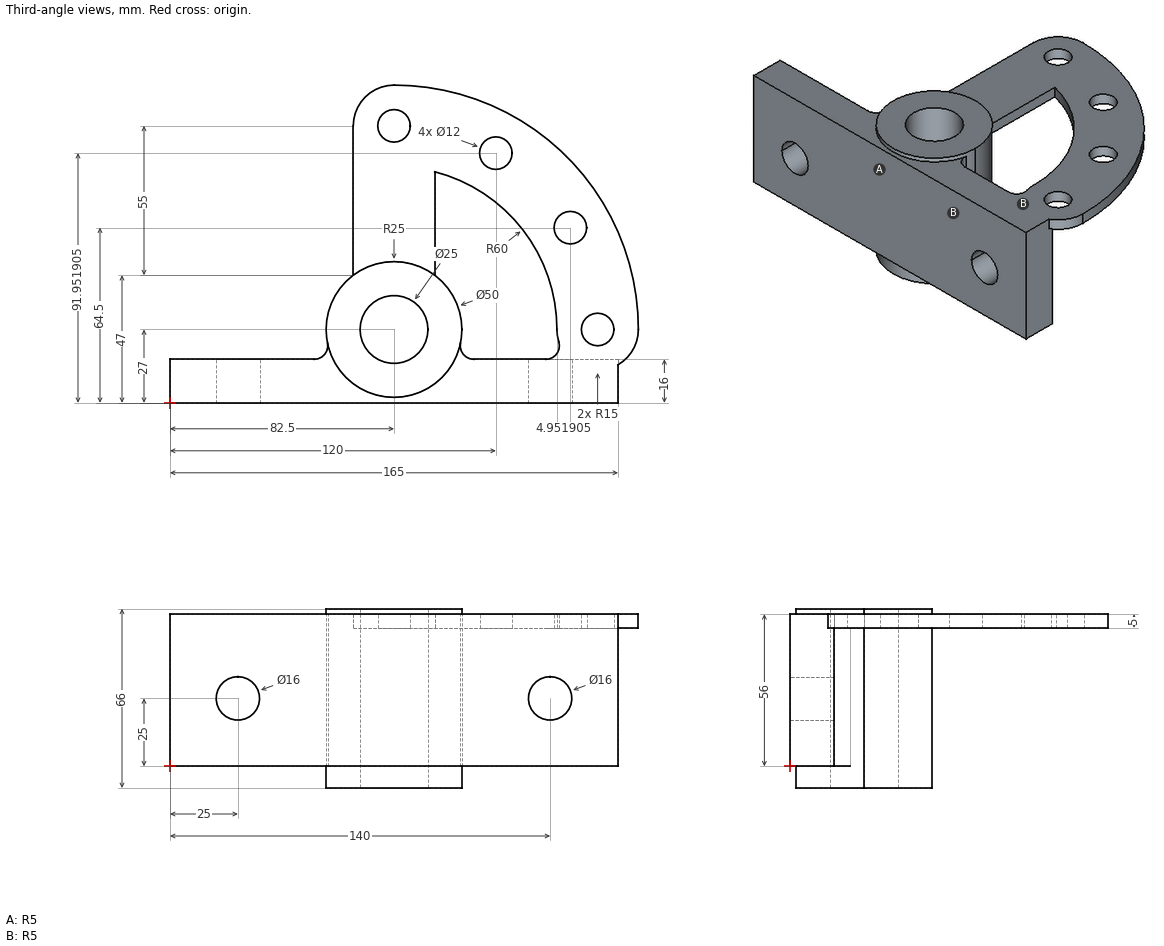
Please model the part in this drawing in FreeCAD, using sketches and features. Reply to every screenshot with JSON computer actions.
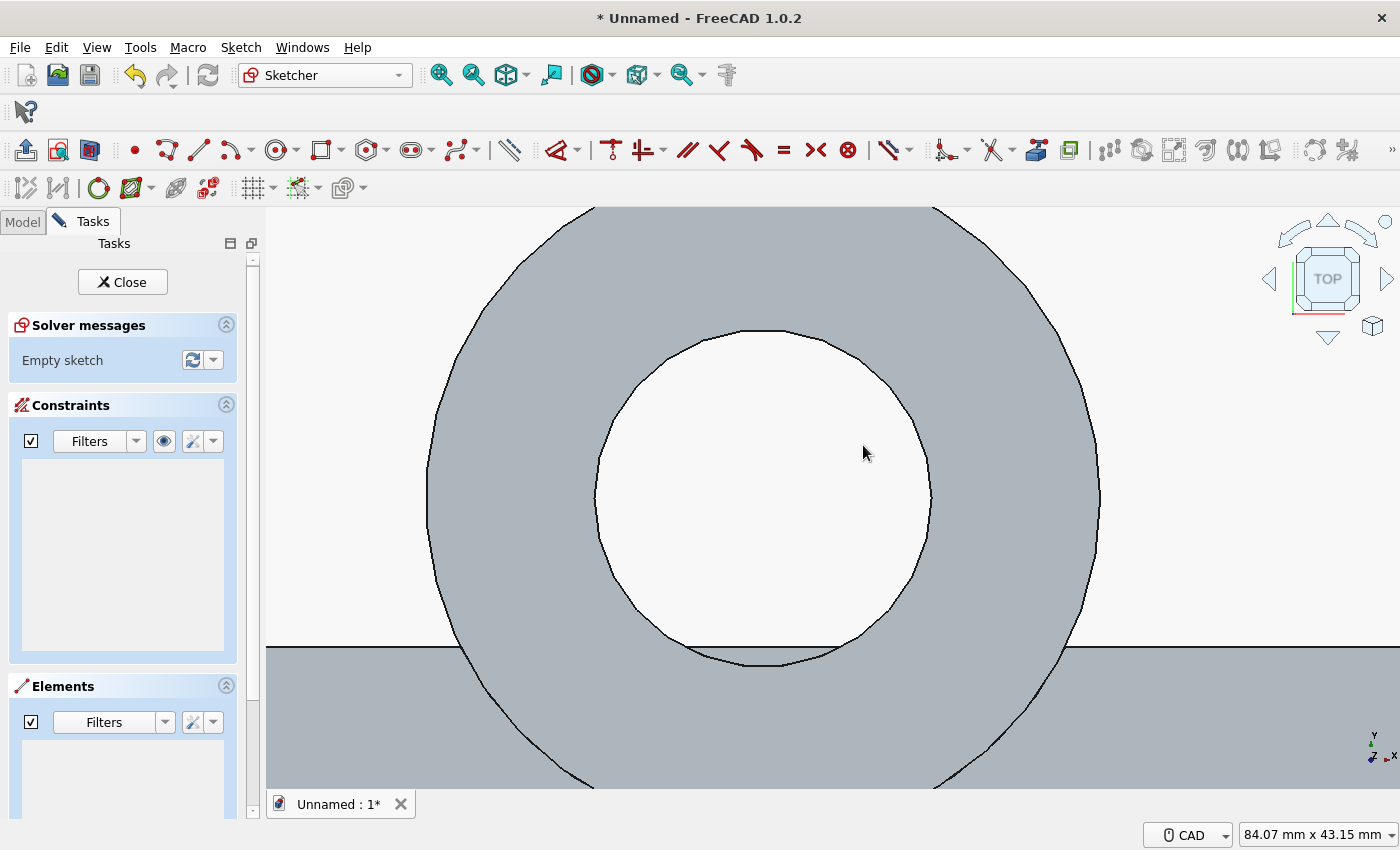
{"action": "left_click", "coordinate": [276, 150]}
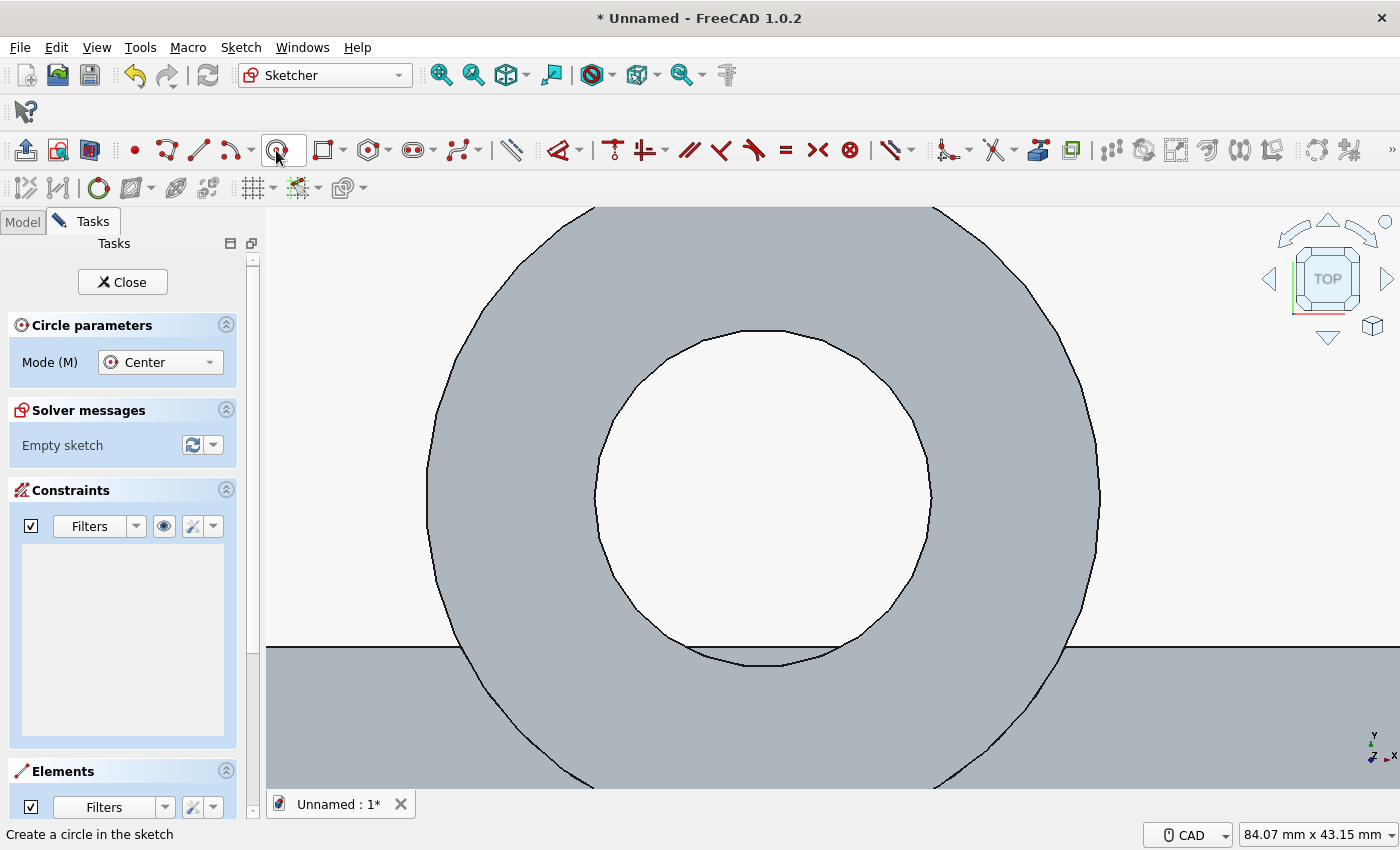
{"action": "left_click", "coordinate": [763, 498]}
{"action": "left_click", "coordinate": [882, 379]}
{"action": "key", "text": "Escape"}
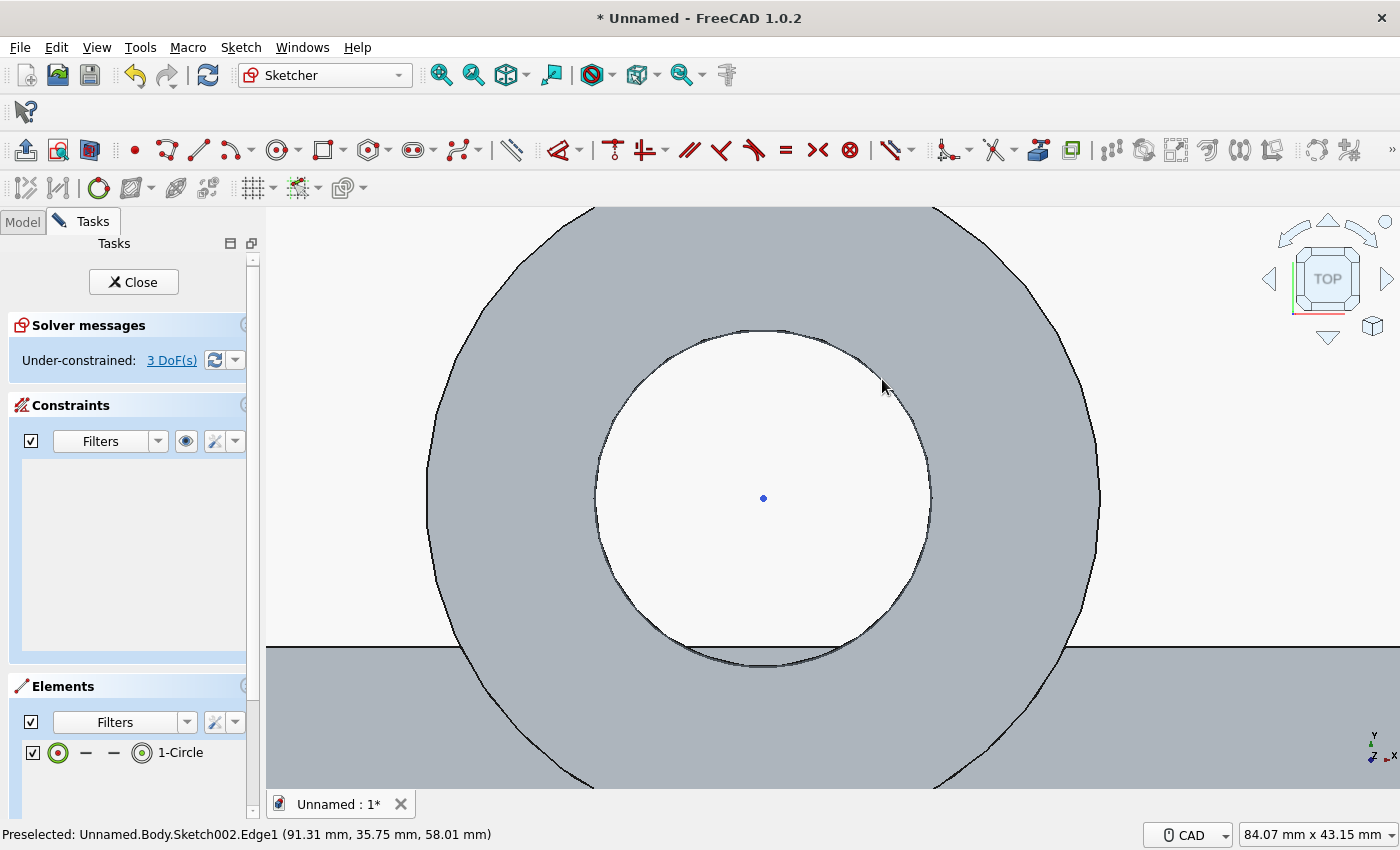
{"action": "left_click", "coordinate": [558, 150]}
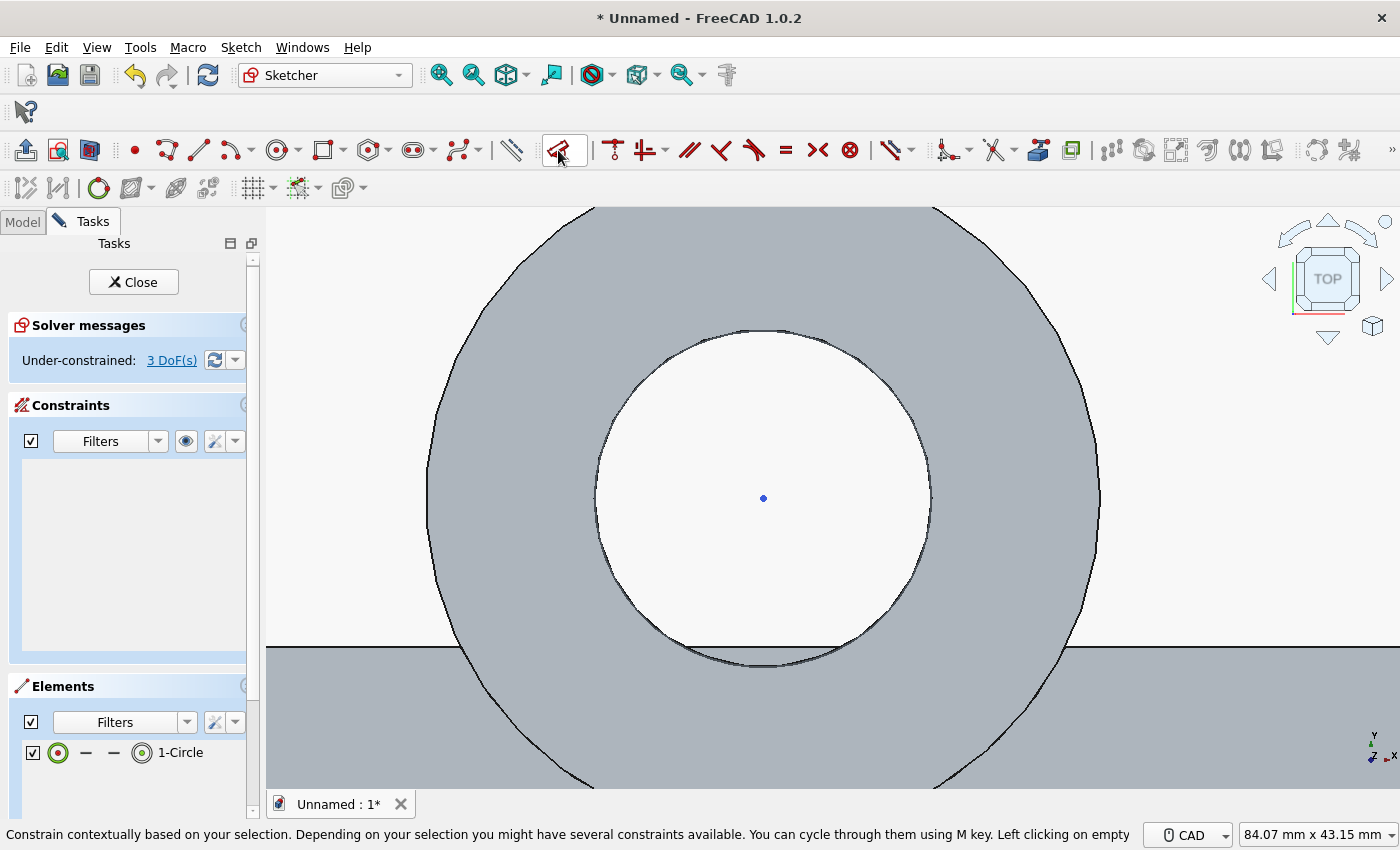
{"action": "left_click", "coordinate": [882, 380]}
{"action": "left_click", "coordinate": [905, 357]}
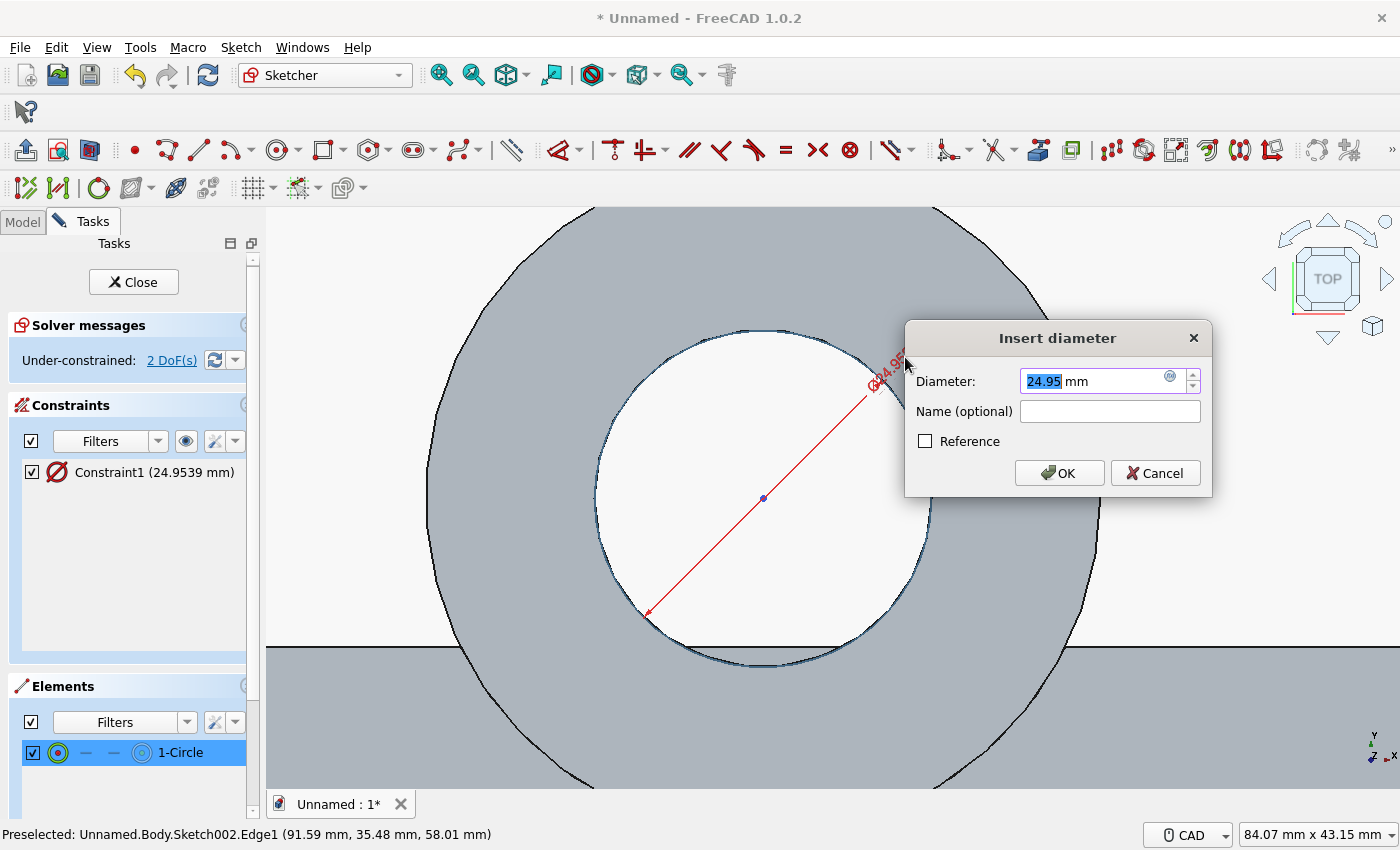
{"action": "type", "text": "25"}
{"action": "key", "text": "Return"}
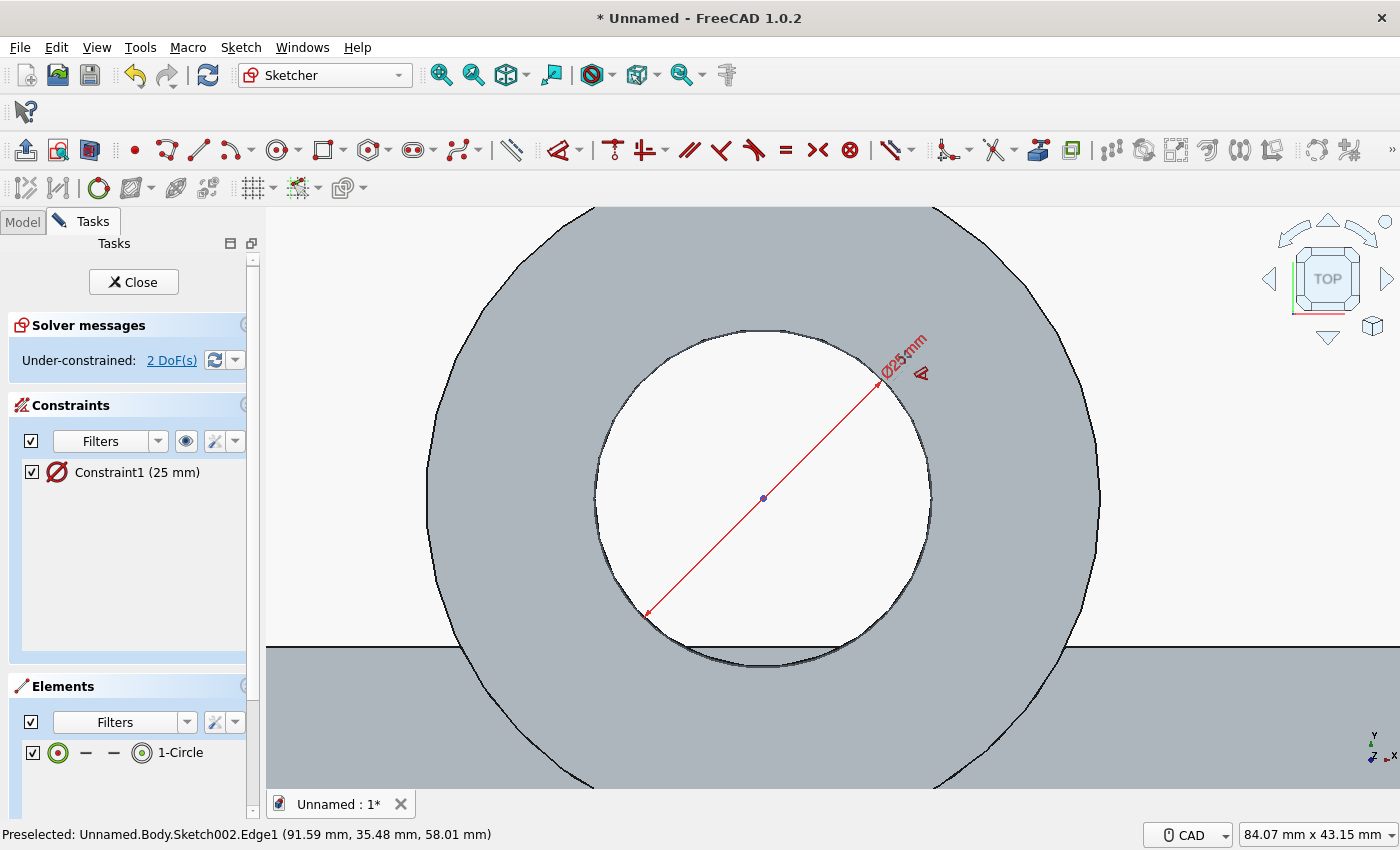
{"action": "left_click", "coordinate": [763, 499]}
{"action": "left_click", "coordinate": [797, 630]}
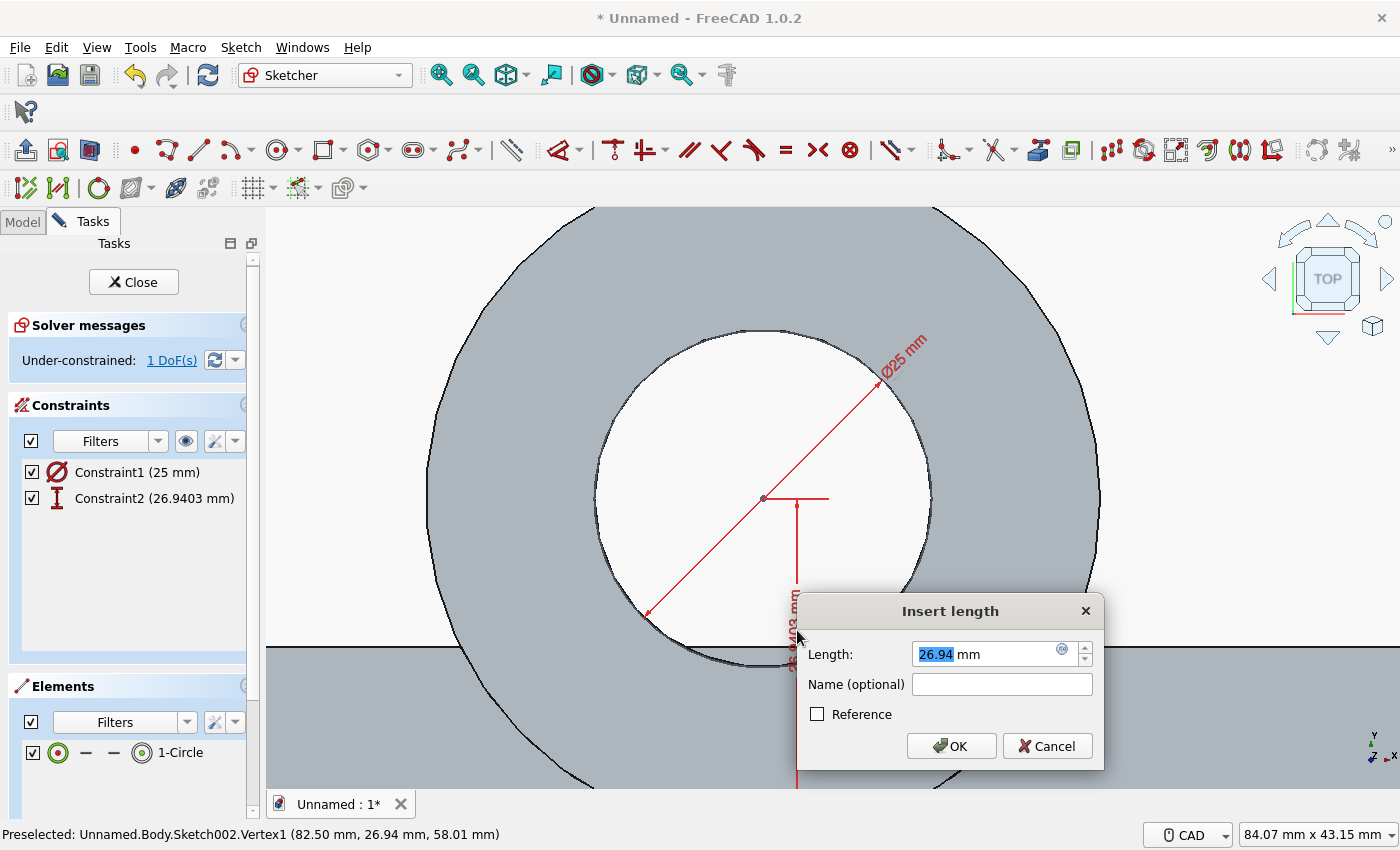
{"action": "type", "text": "27"}
{"action": "key", "text": "Return"}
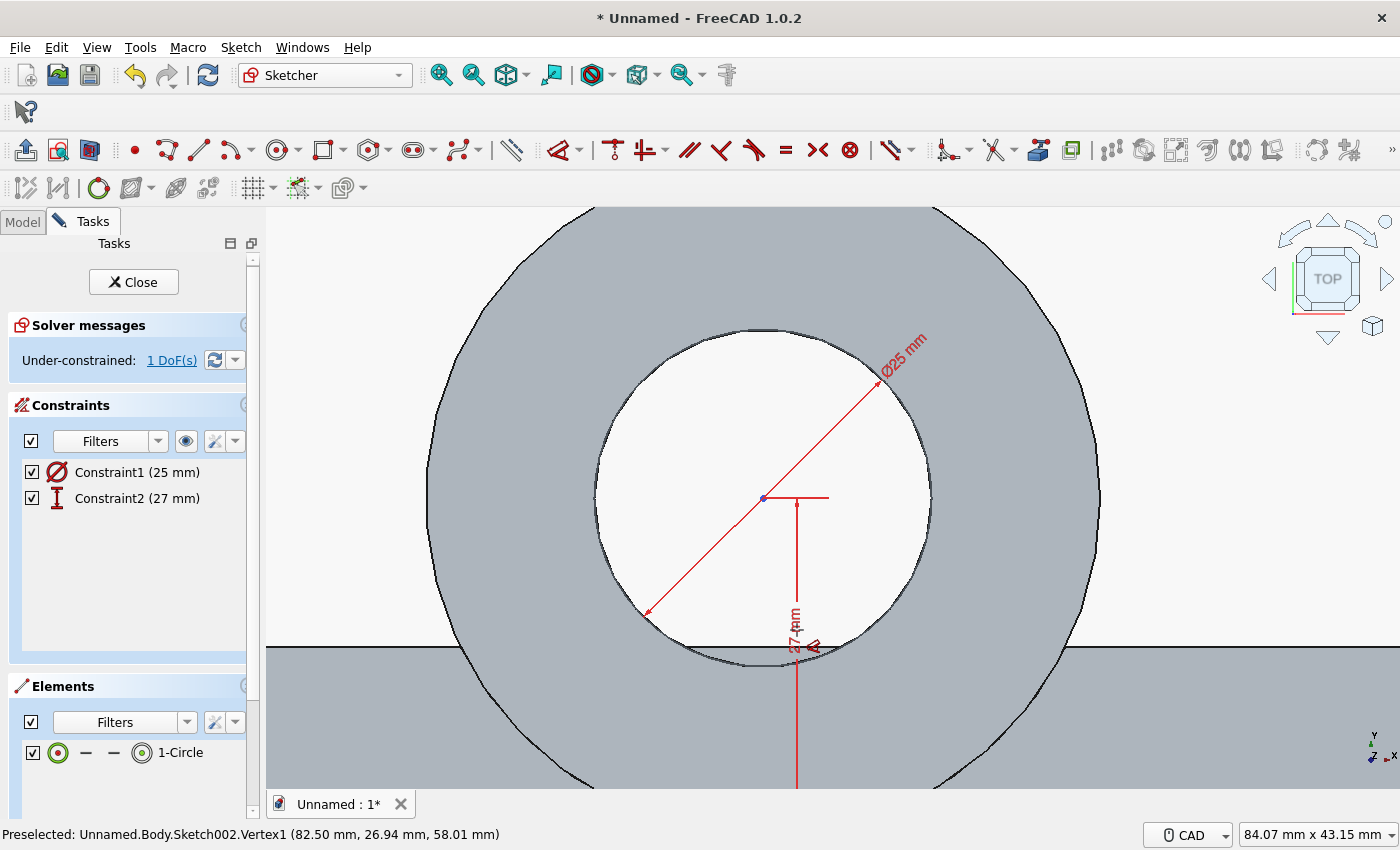
{"action": "left_click", "coordinate": [763, 498]}
{"action": "left_click", "coordinate": [529, 464]}